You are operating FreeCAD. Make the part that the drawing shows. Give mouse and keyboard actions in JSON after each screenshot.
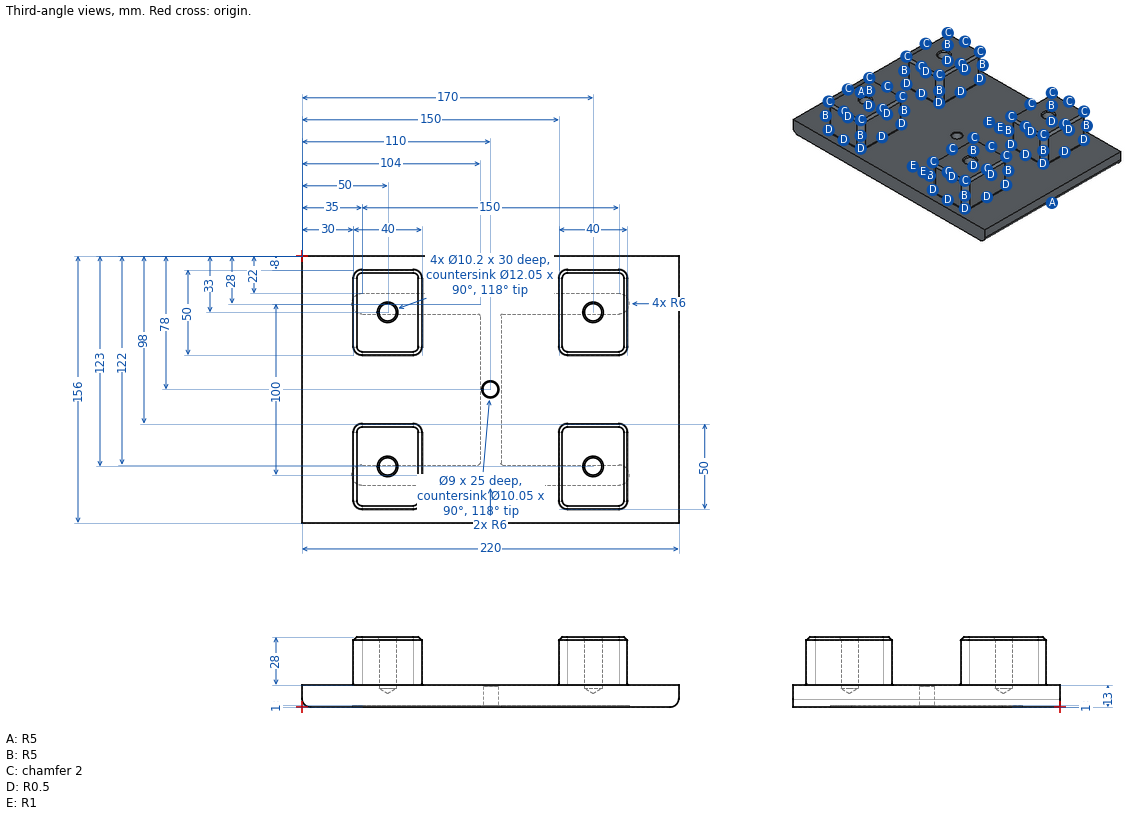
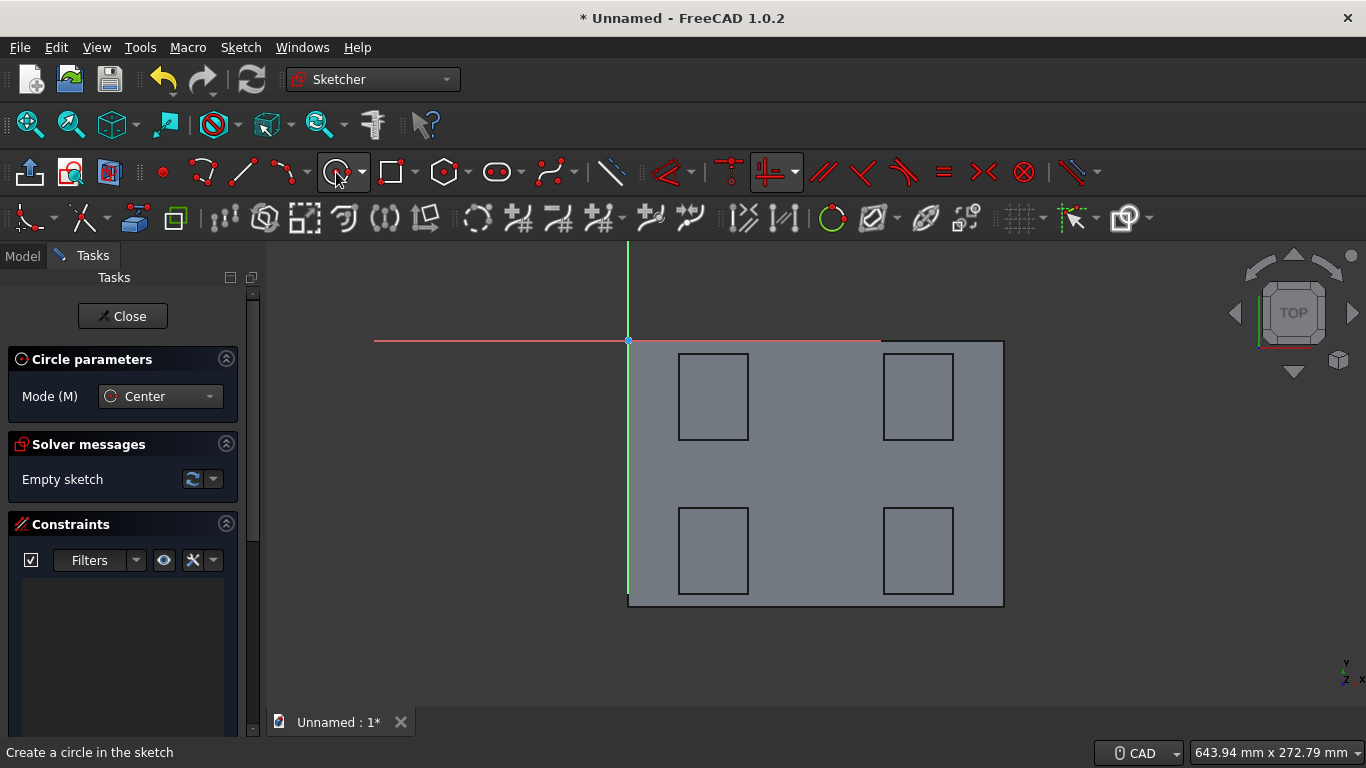
{"action": "scroll", "coordinate": [714, 397], "scroll_direction": "up", "scroll_amount": 5}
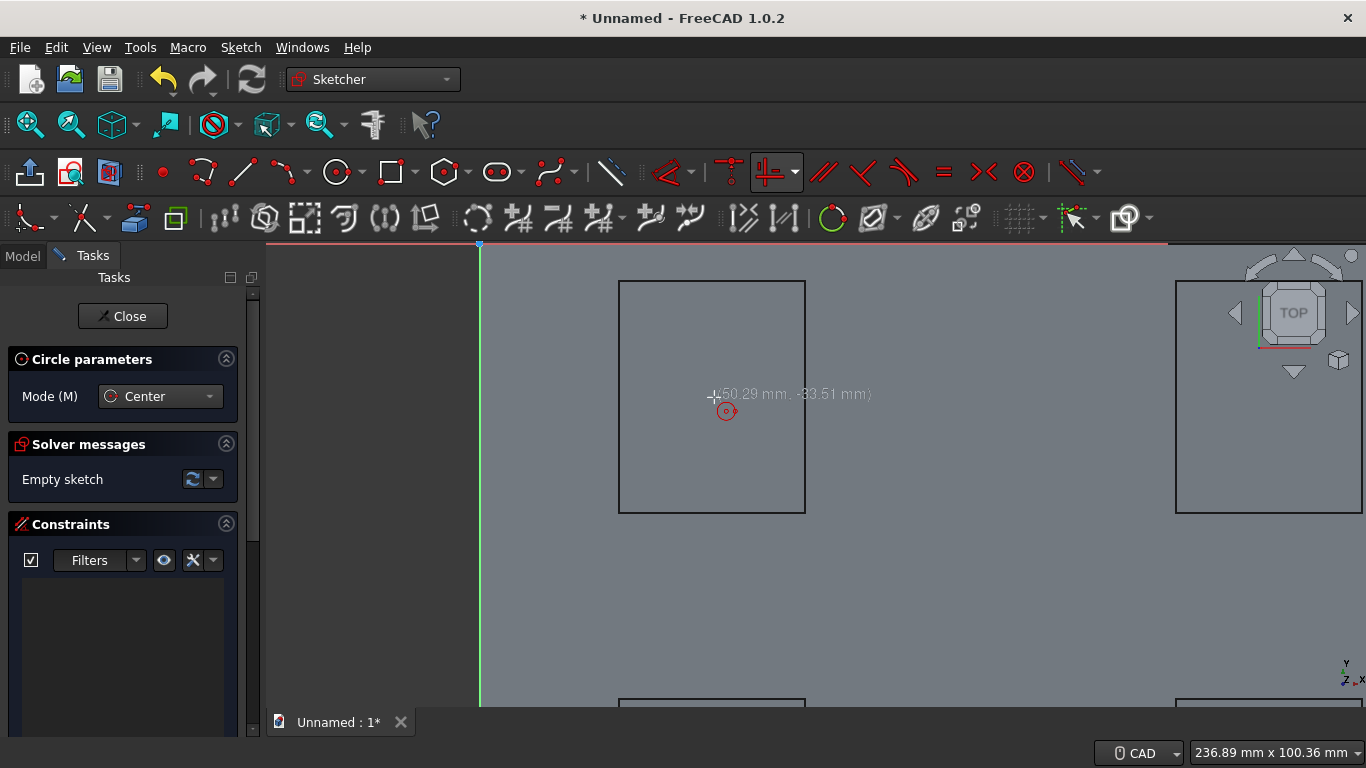
{"action": "left_click", "coordinate": [712, 397]}
{"action": "left_click", "coordinate": [729, 380]}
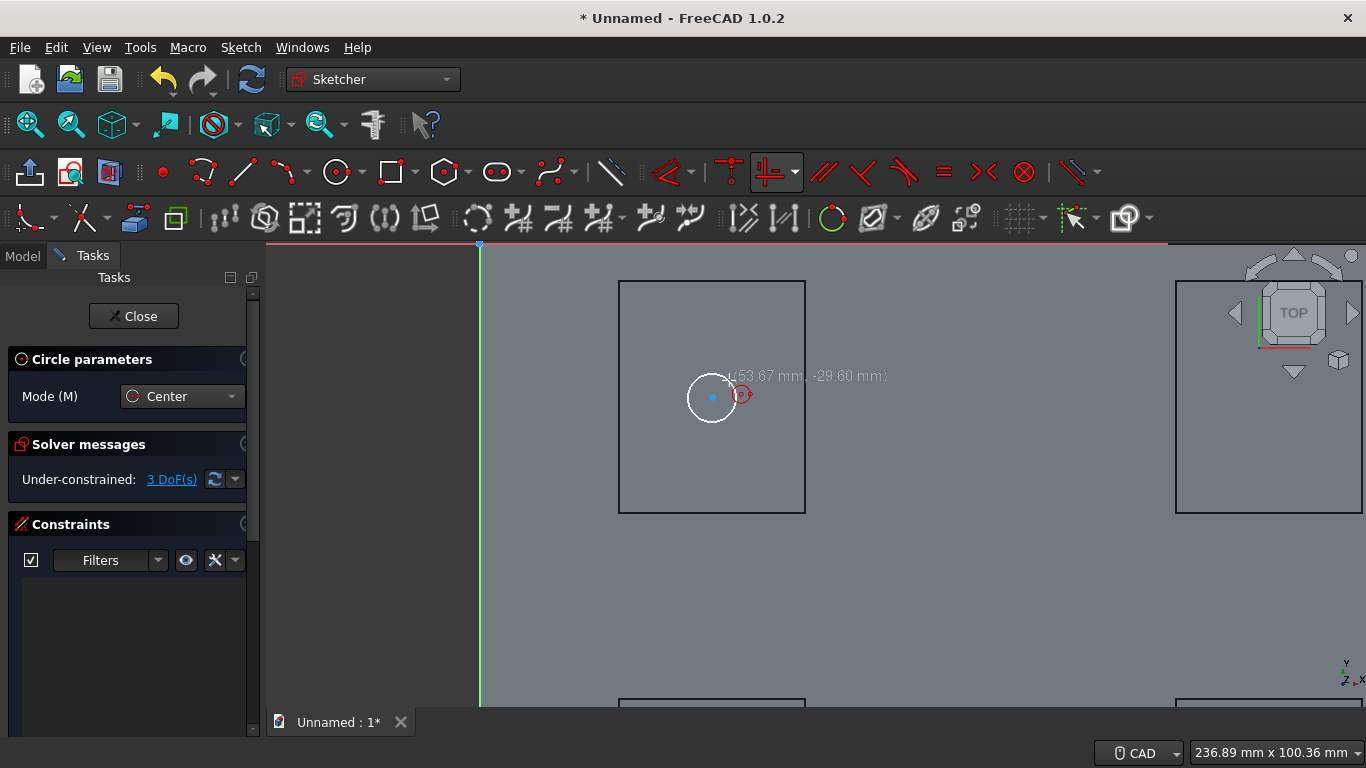
{"action": "scroll", "coordinate": [634, 419], "scroll_direction": "down", "scroll_amount": 4}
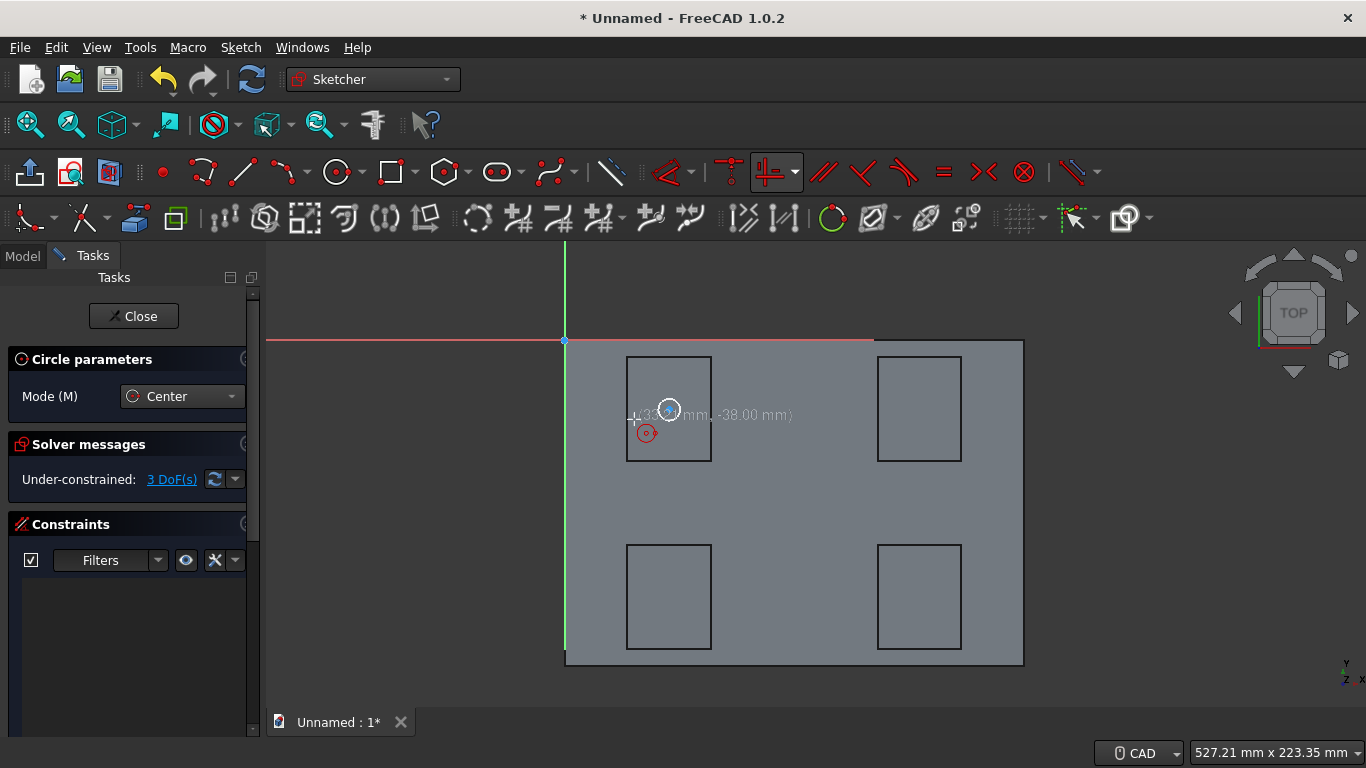
{"action": "scroll", "coordinate": [920, 409], "scroll_direction": "up", "scroll_amount": 4}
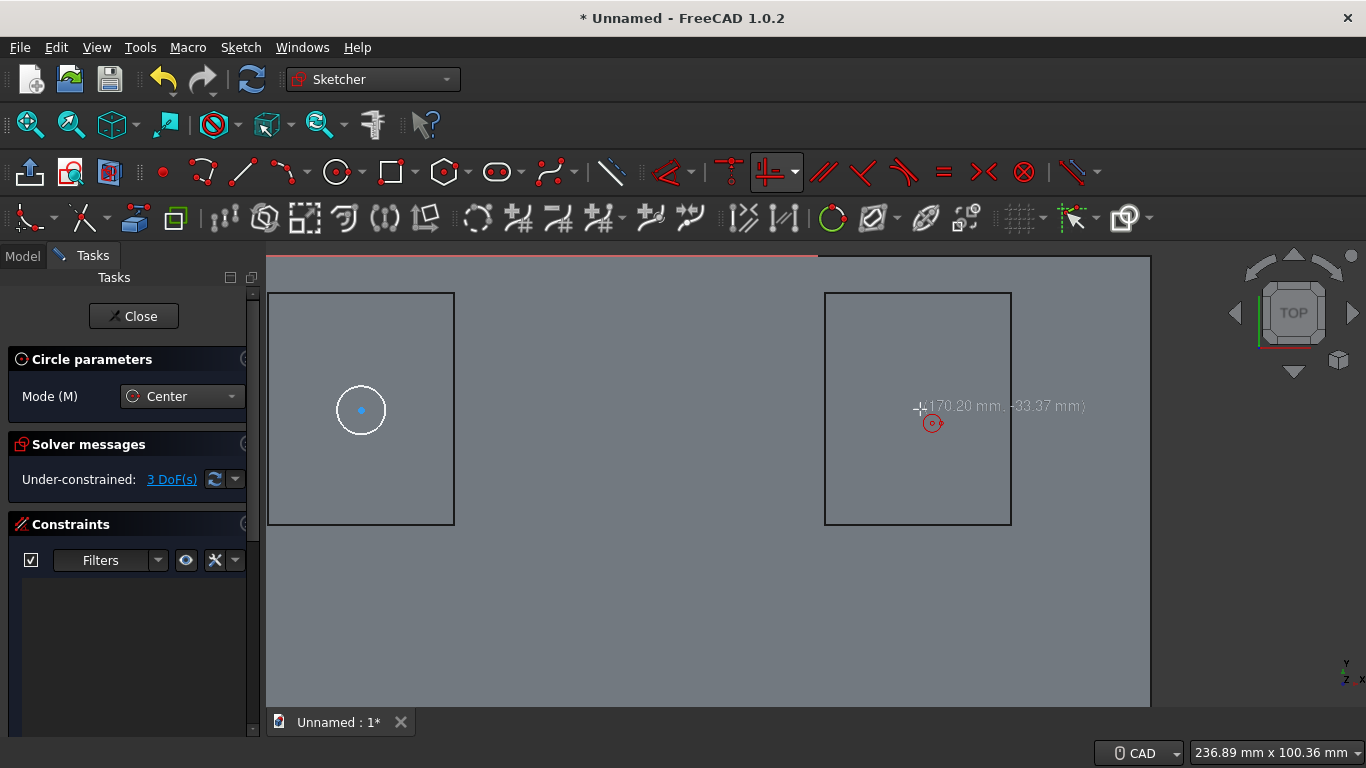
{"action": "left_click", "coordinate": [918, 409]}
{"action": "left_click", "coordinate": [935, 392]}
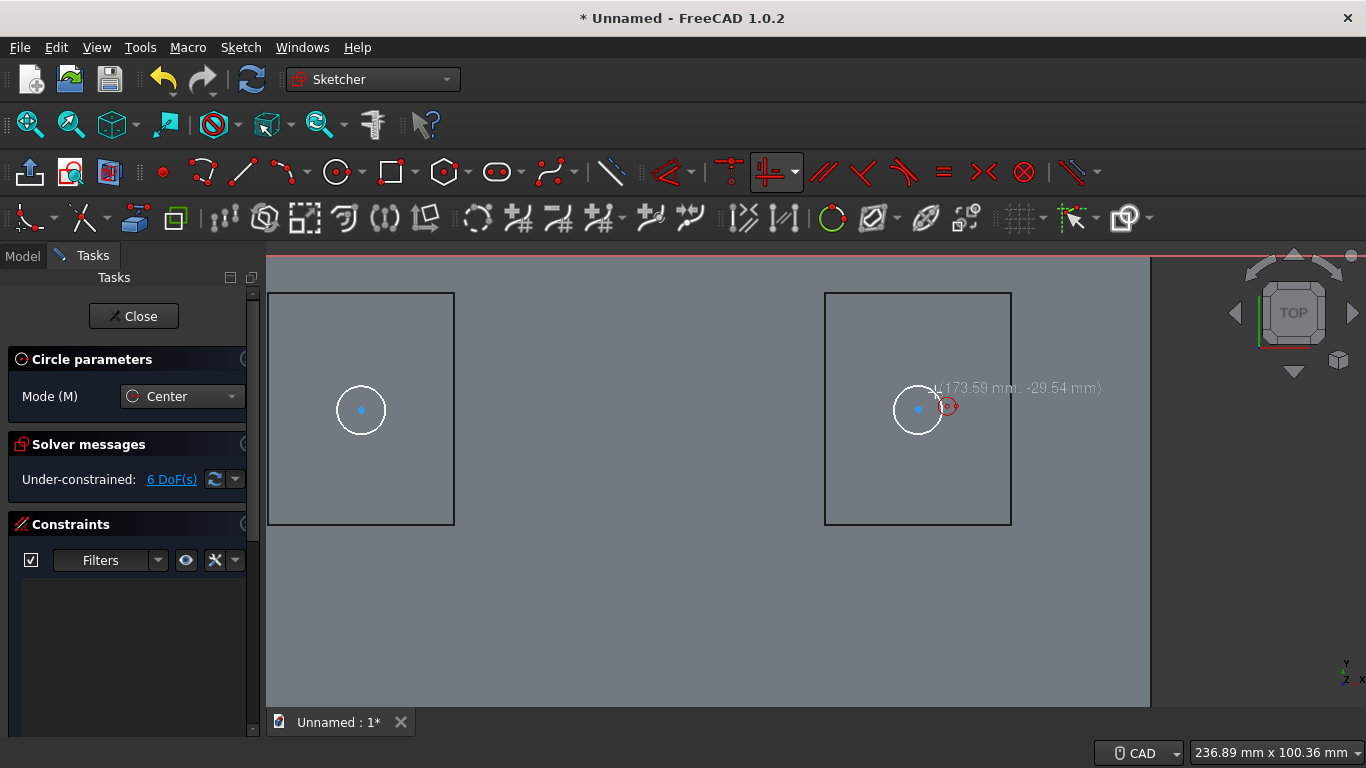
{"action": "scroll", "coordinate": [920, 409], "scroll_direction": "down", "scroll_amount": 4}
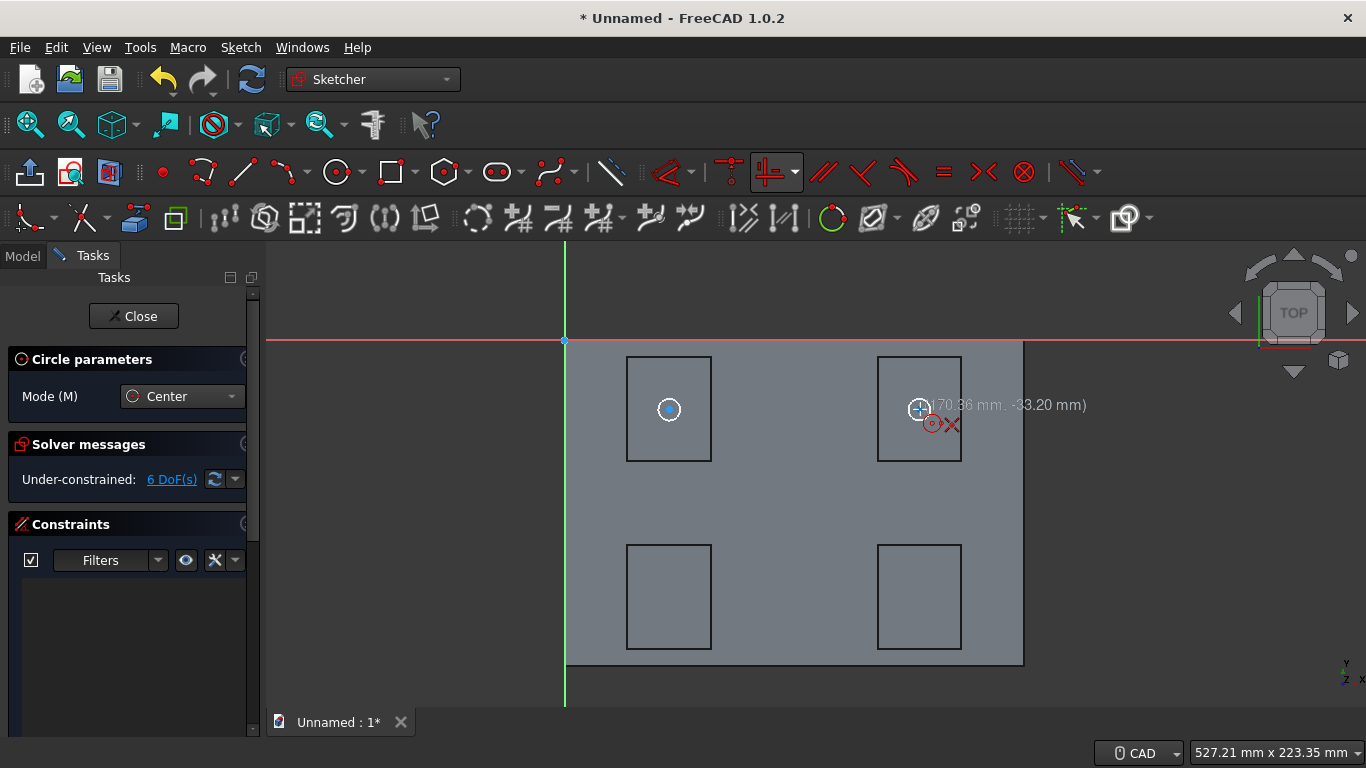
{"action": "scroll", "coordinate": [920, 597], "scroll_direction": "up", "scroll_amount": 4}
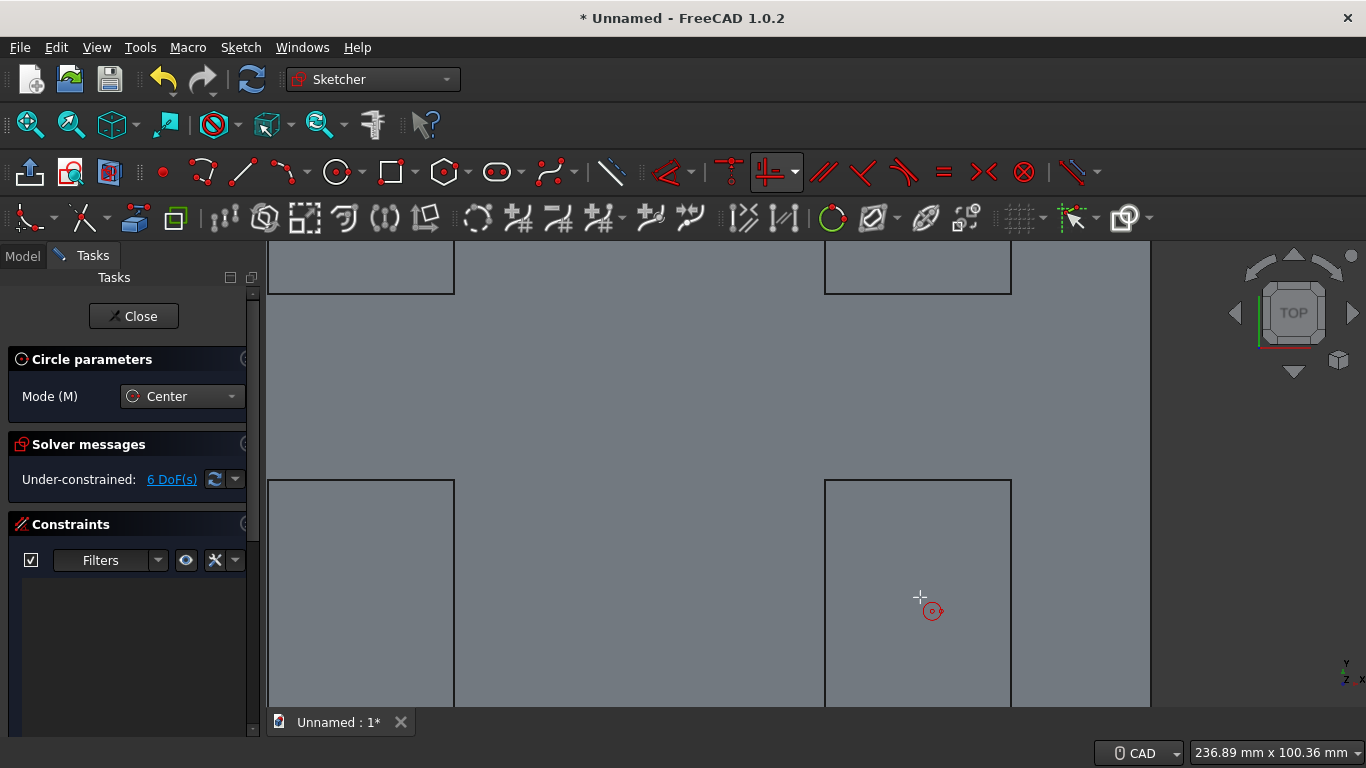
{"action": "left_click", "coordinate": [918, 596]}
{"action": "left_click", "coordinate": [935, 579]}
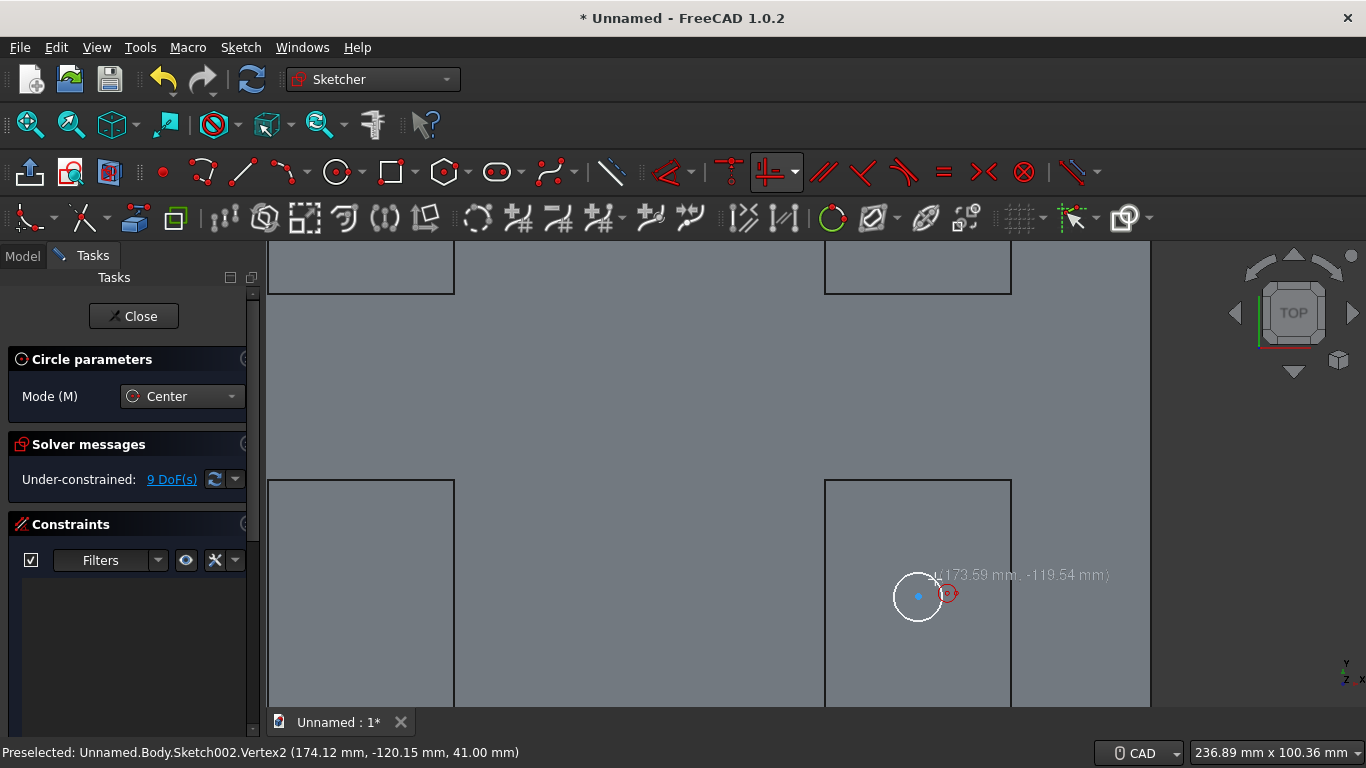
{"action": "left_click", "coordinate": [361, 596]}
{"action": "left_click", "coordinate": [378, 579]}
{"action": "key", "text": "Escape"}